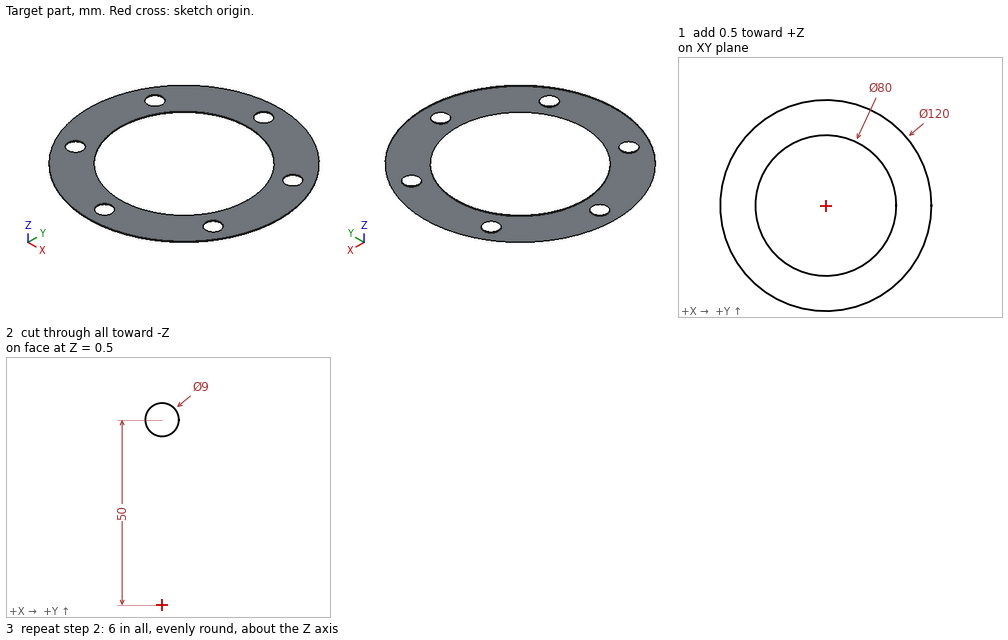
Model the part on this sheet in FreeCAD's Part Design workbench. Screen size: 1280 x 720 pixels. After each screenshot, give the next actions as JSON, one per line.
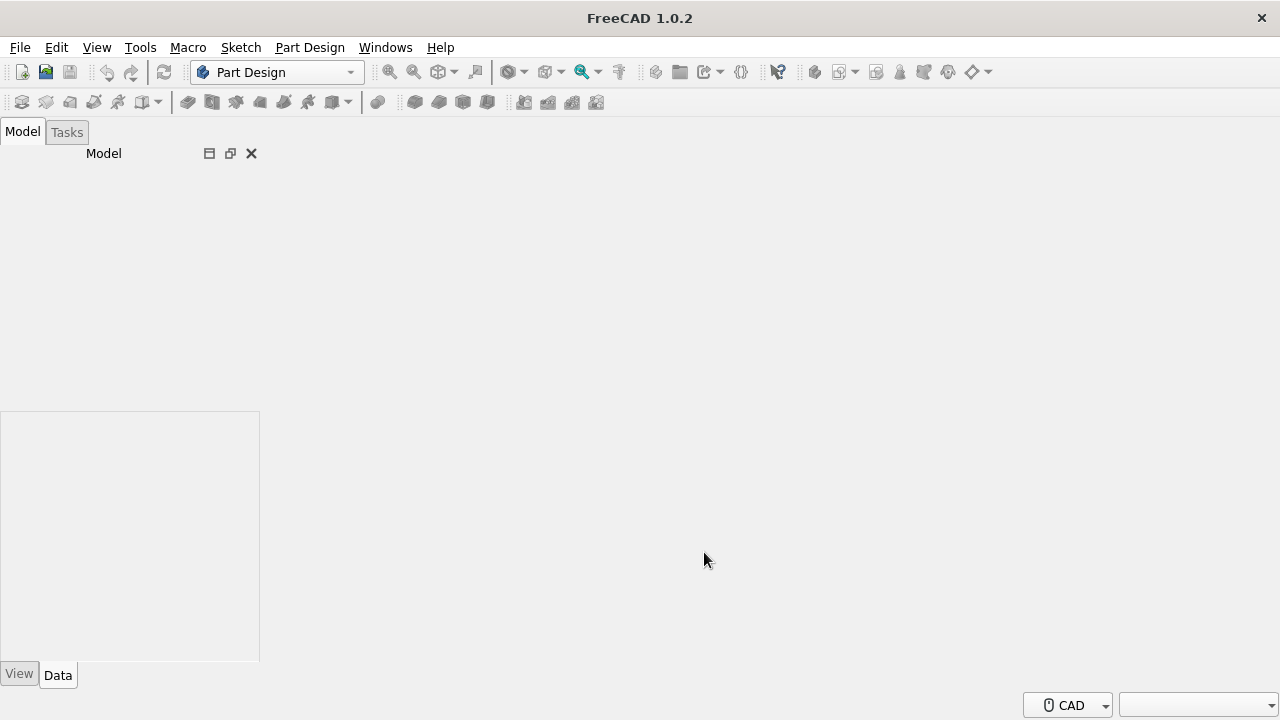
{"action": "left_click", "coordinate": [22, 72]}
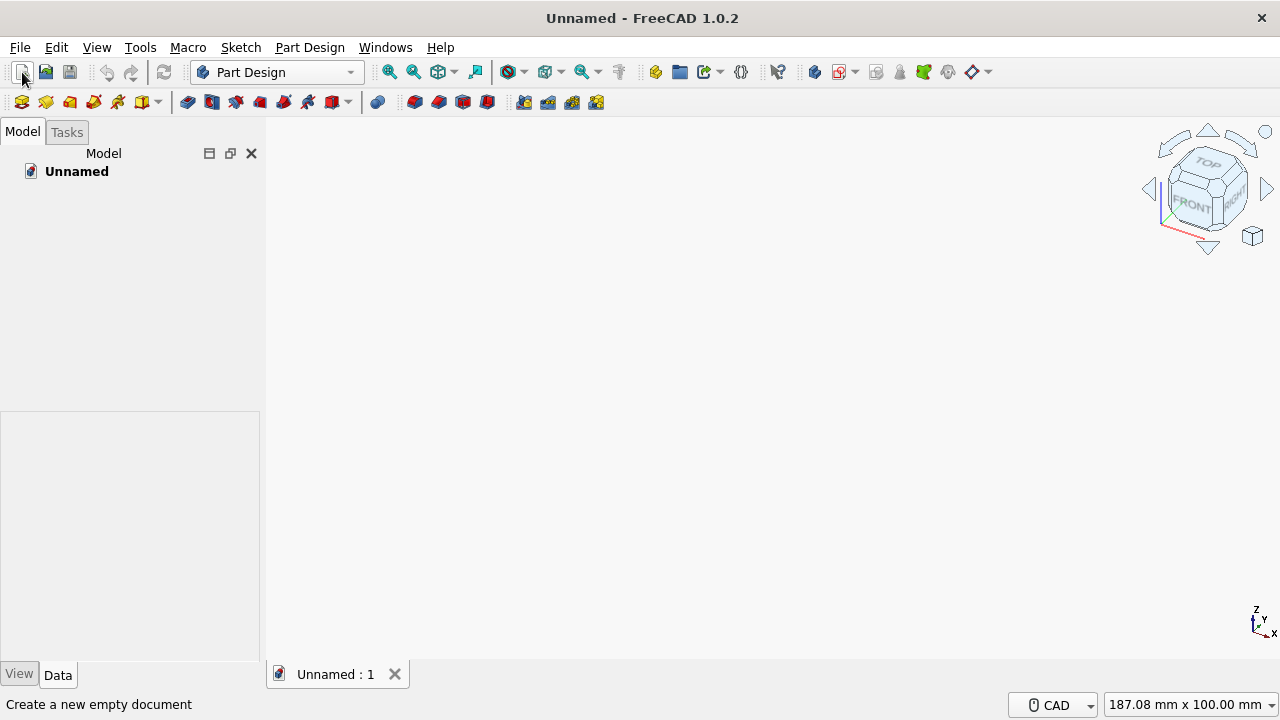
{"action": "left_click", "coordinate": [840, 72]}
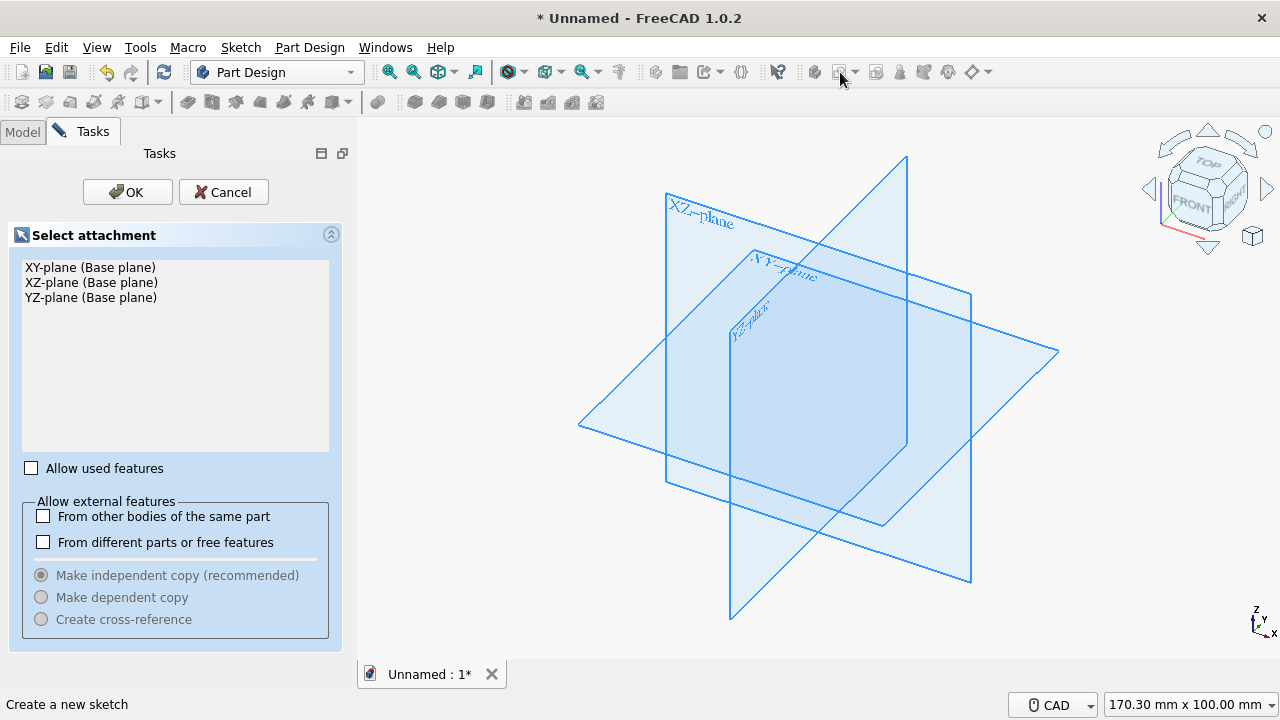
{"action": "left_click", "coordinate": [82, 268]}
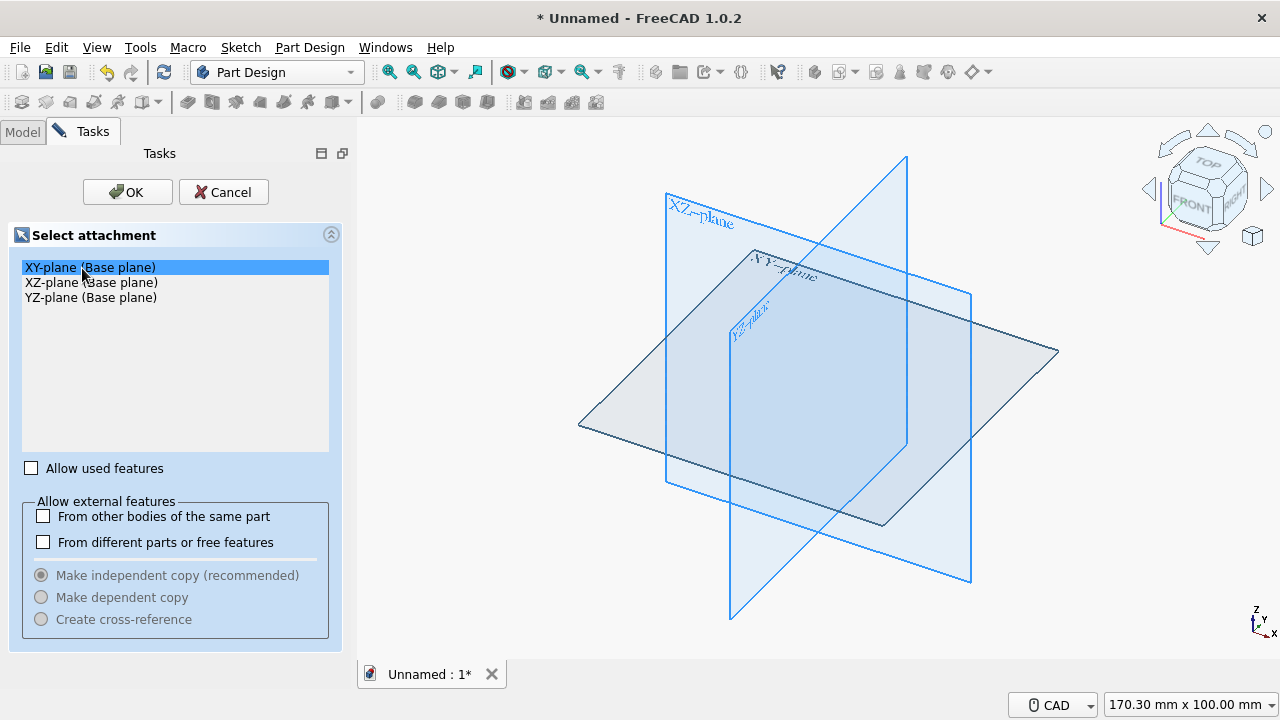
{"action": "left_click", "coordinate": [128, 192]}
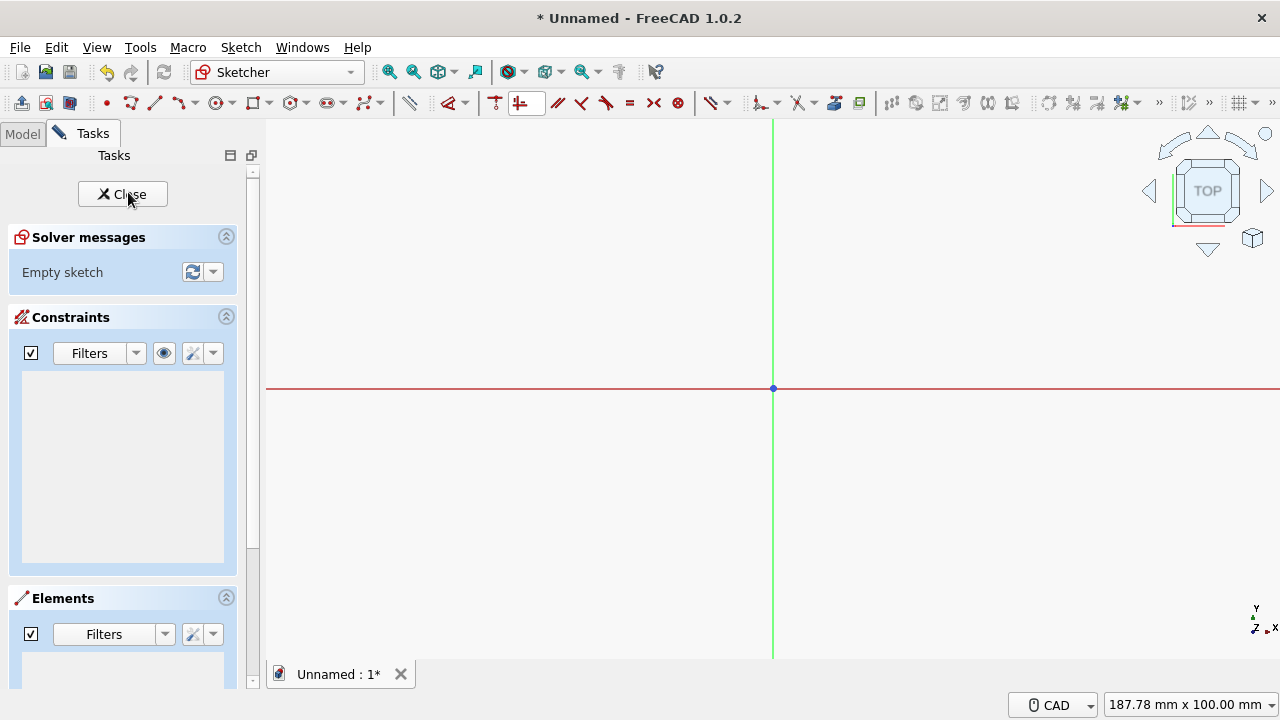
{"action": "scroll", "coordinate": [621, 389], "scroll_direction": "down", "scroll_amount": 3}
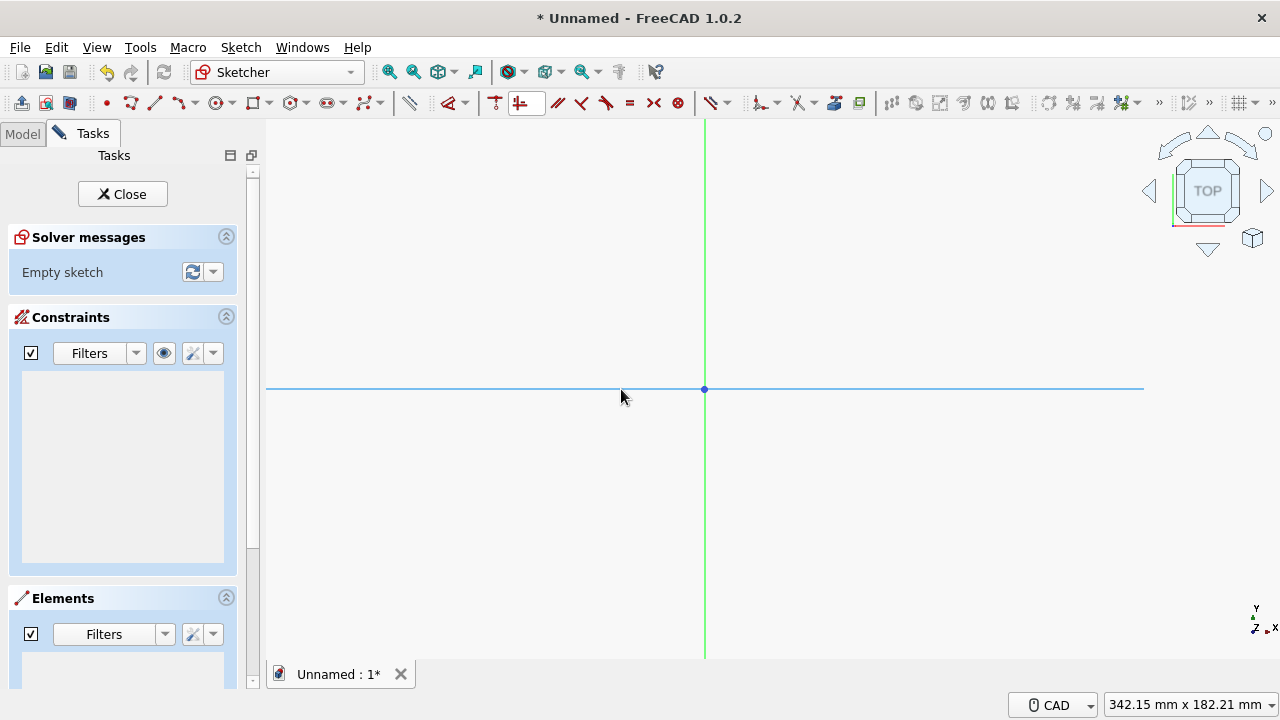
{"action": "key", "text": "g c"}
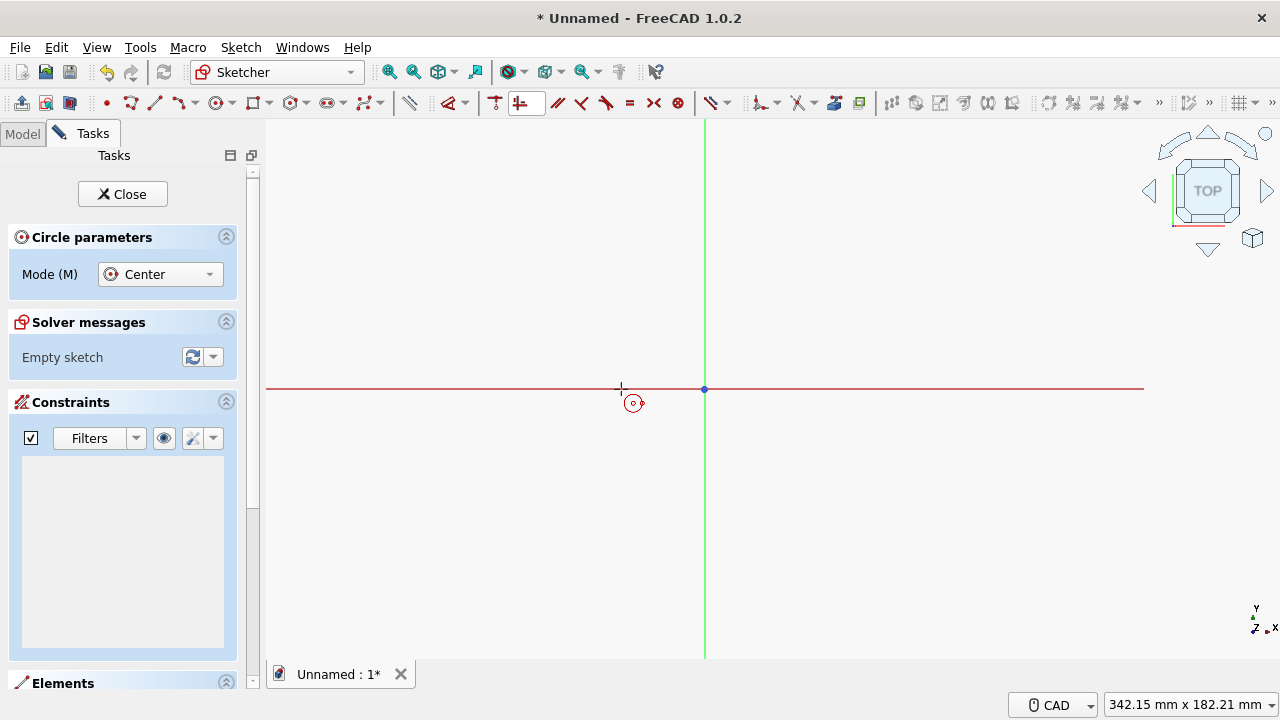
{"action": "left_click", "coordinate": [705, 389]}
{"action": "mouse_move", "coordinate": [830, 263]}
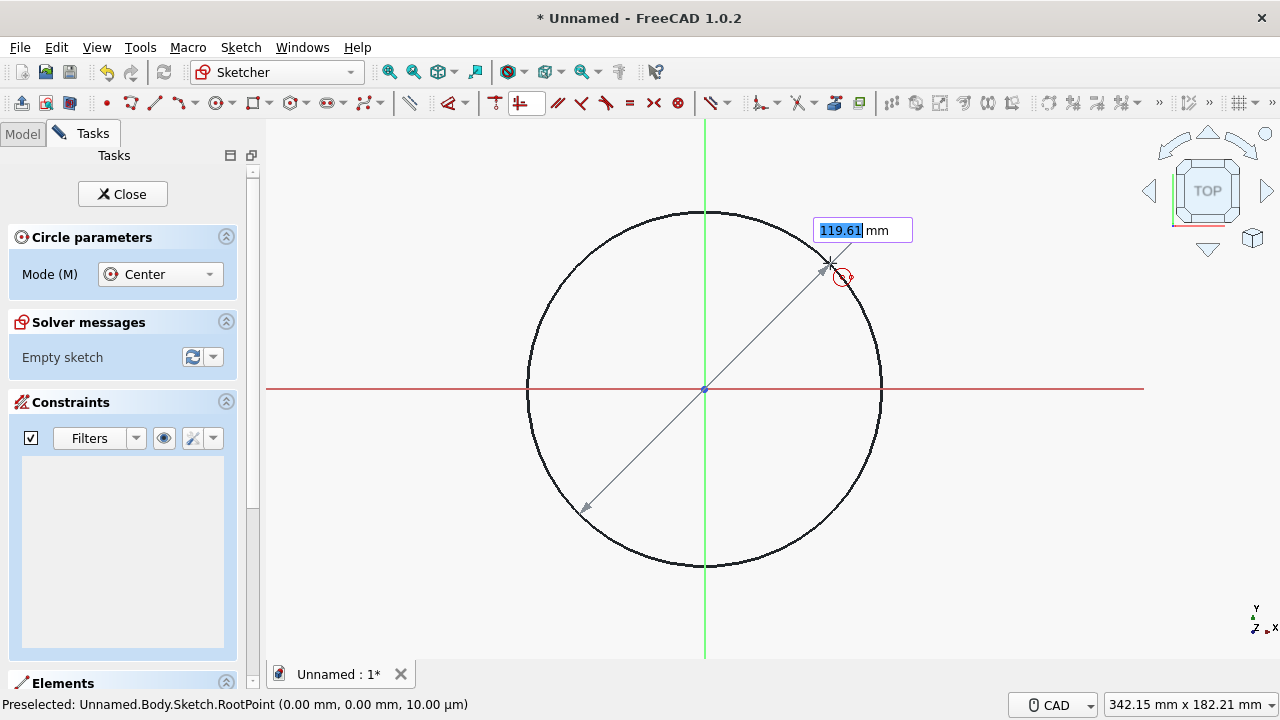
{"action": "type", "text": "120"}
{"action": "key", "text": "Return"}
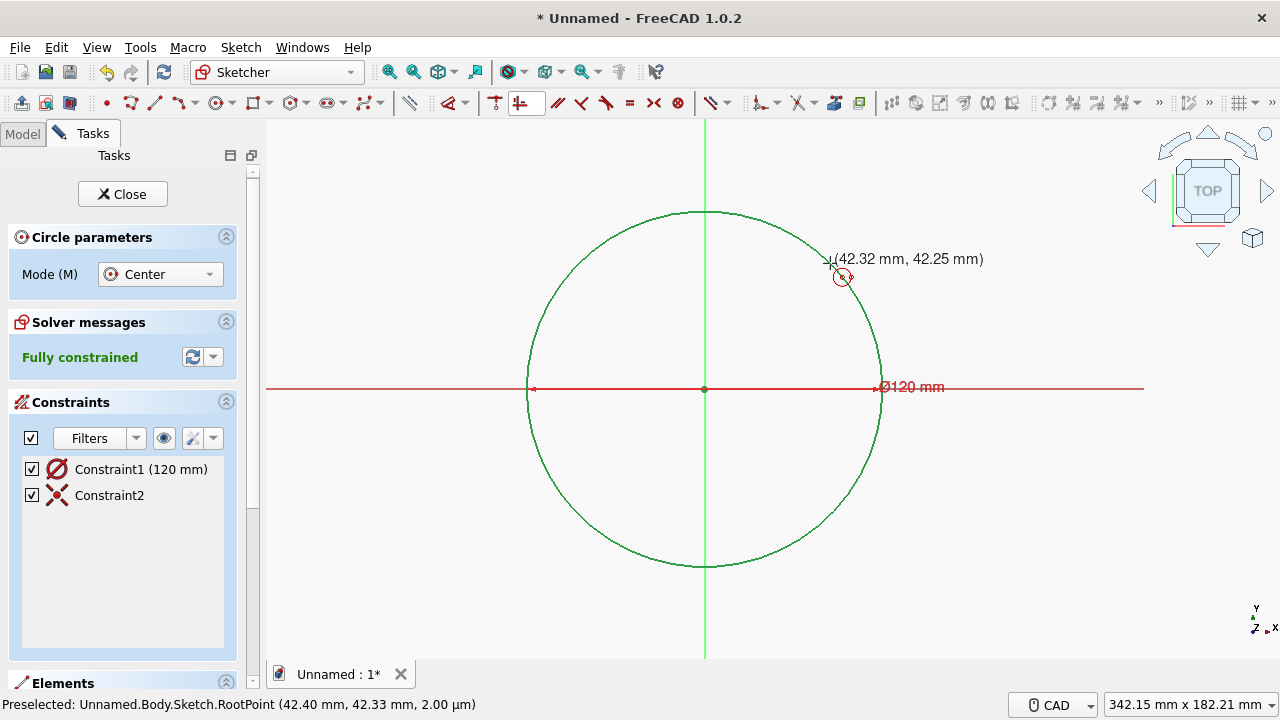
{"action": "left_click", "coordinate": [705, 389]}
{"action": "mouse_move", "coordinate": [788, 305]}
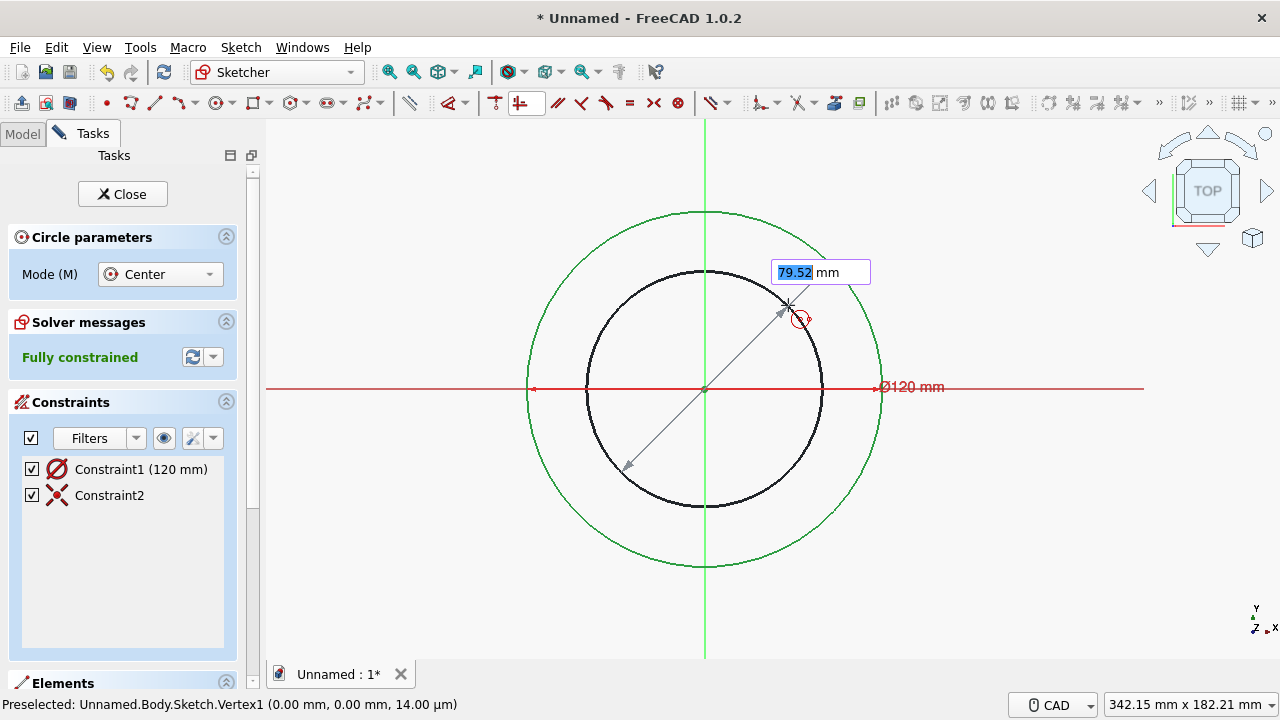
{"action": "type", "text": "80"}
{"action": "key", "text": "Return"}
{"action": "key", "text": "Escape"}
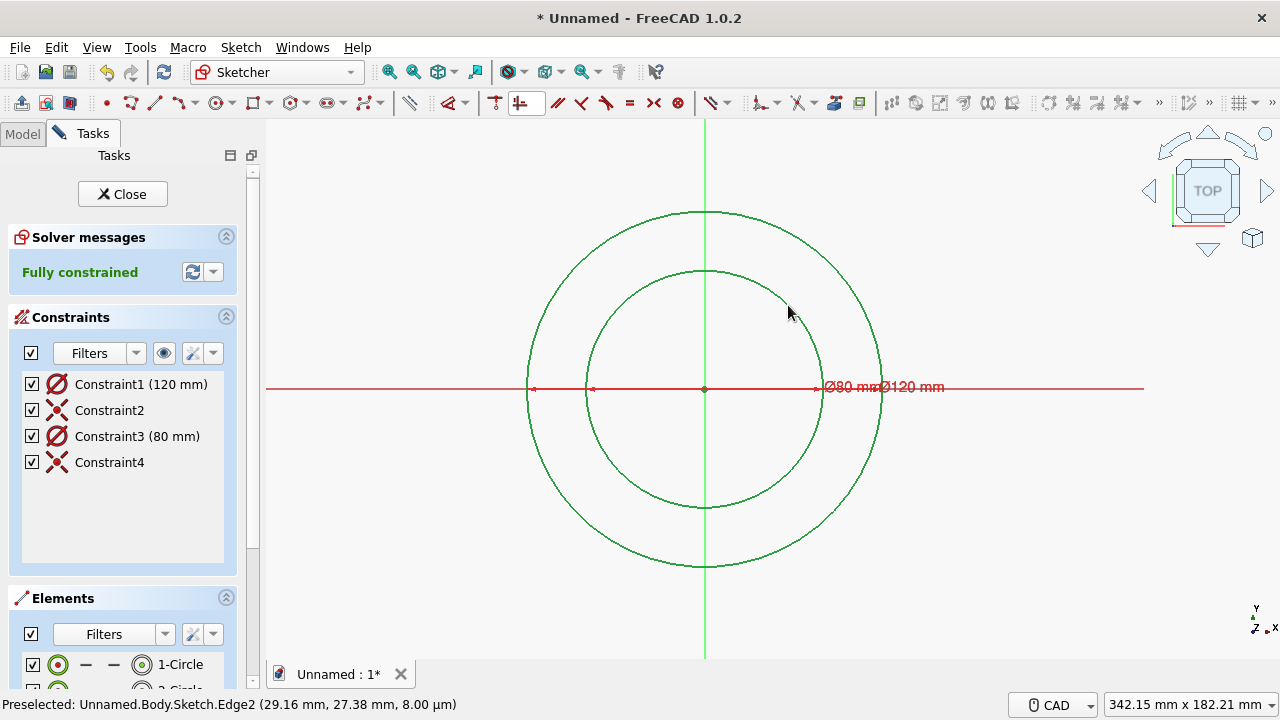
{"action": "left_click", "coordinate": [123, 194]}